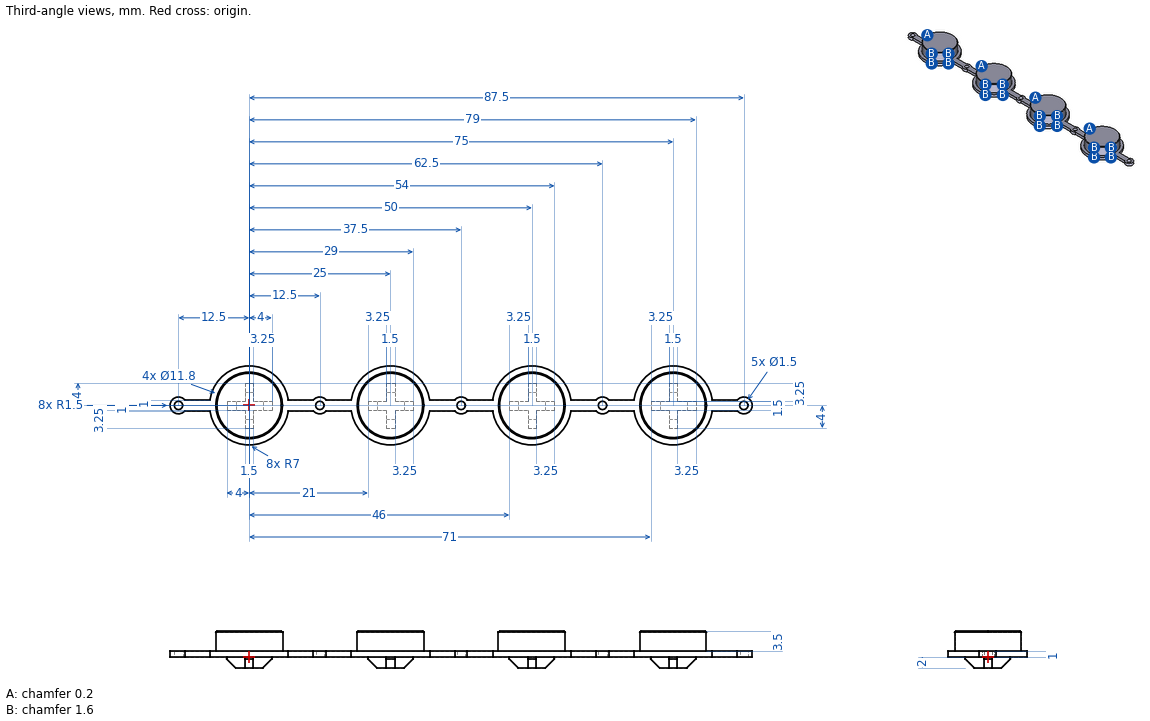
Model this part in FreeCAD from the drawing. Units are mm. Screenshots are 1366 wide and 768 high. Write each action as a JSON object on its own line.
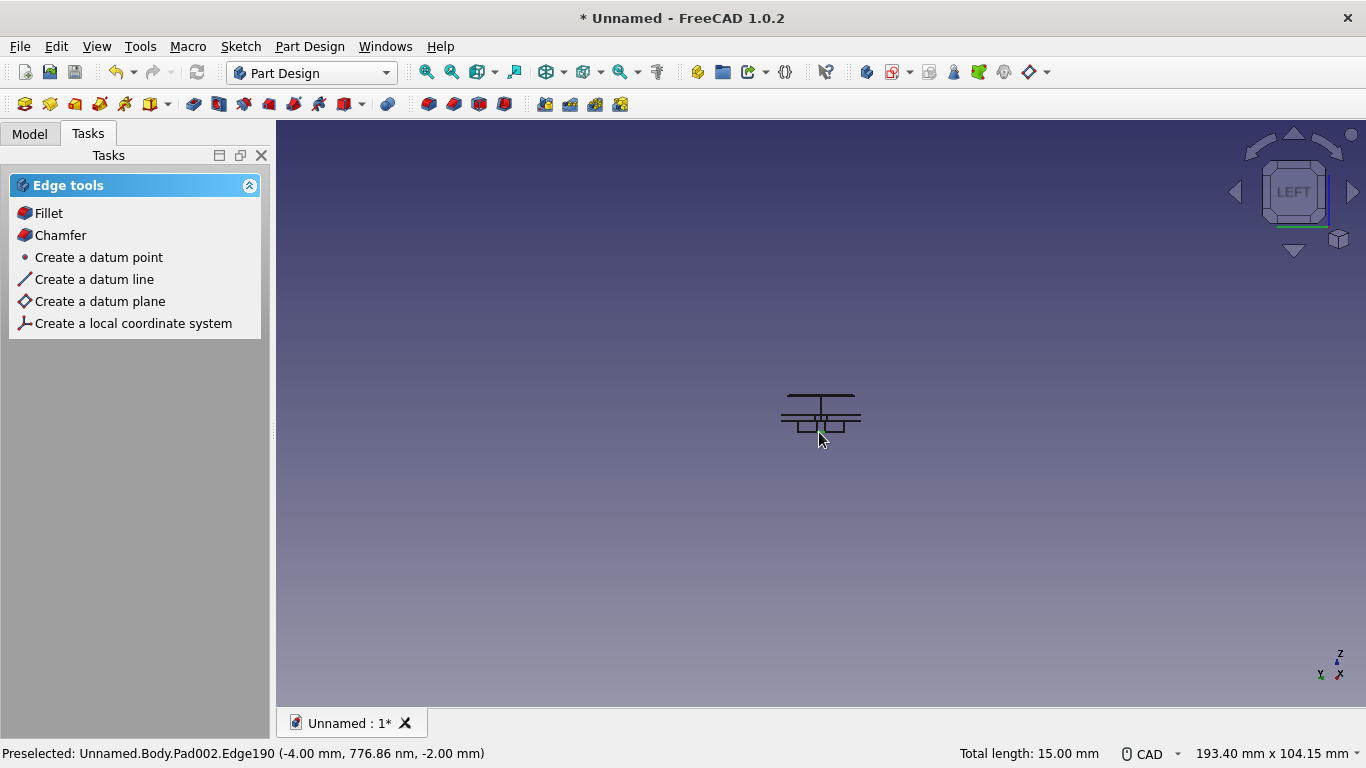
{"action": "key", "text": "0"}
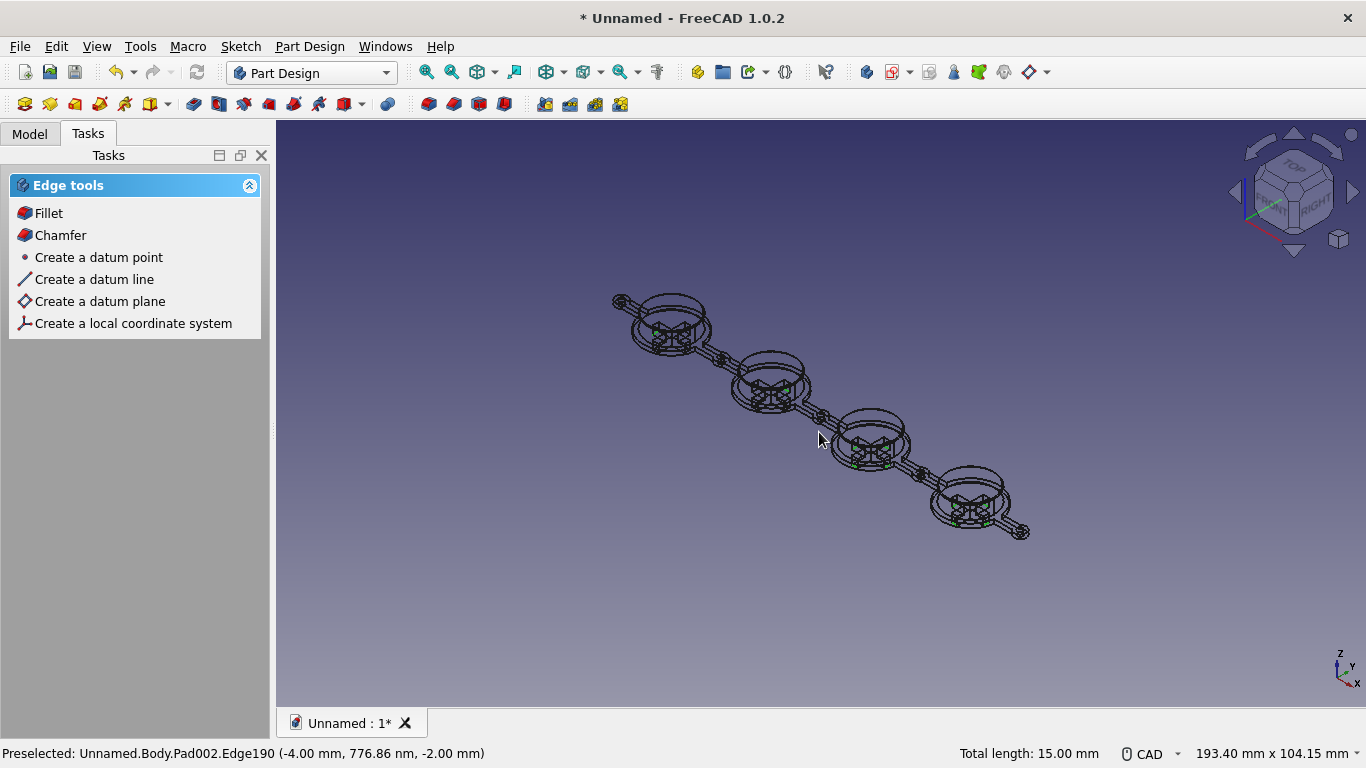
{"action": "scroll", "coordinate": [755, 389], "scroll_direction": "up", "scroll_amount": 8}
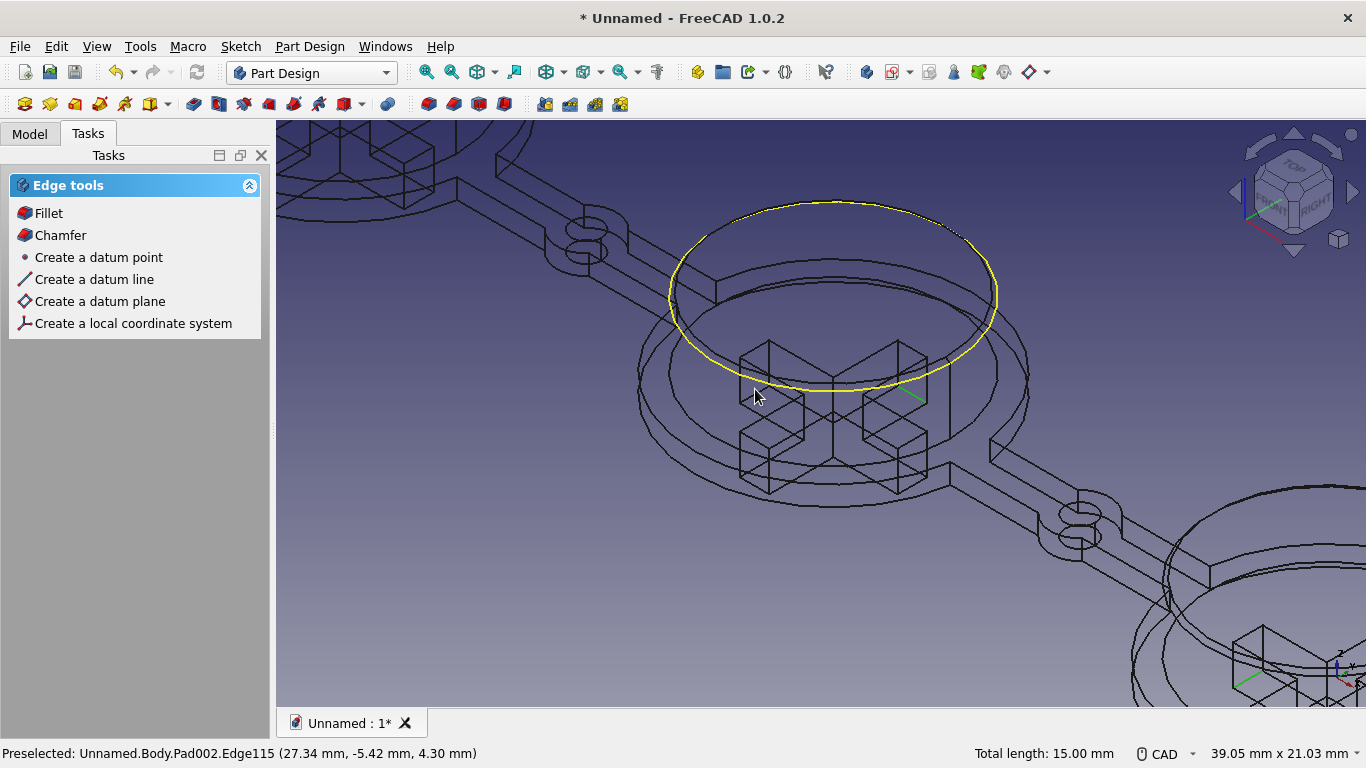
{"action": "left_click", "coordinate": [754, 394], "text": "ctrl"}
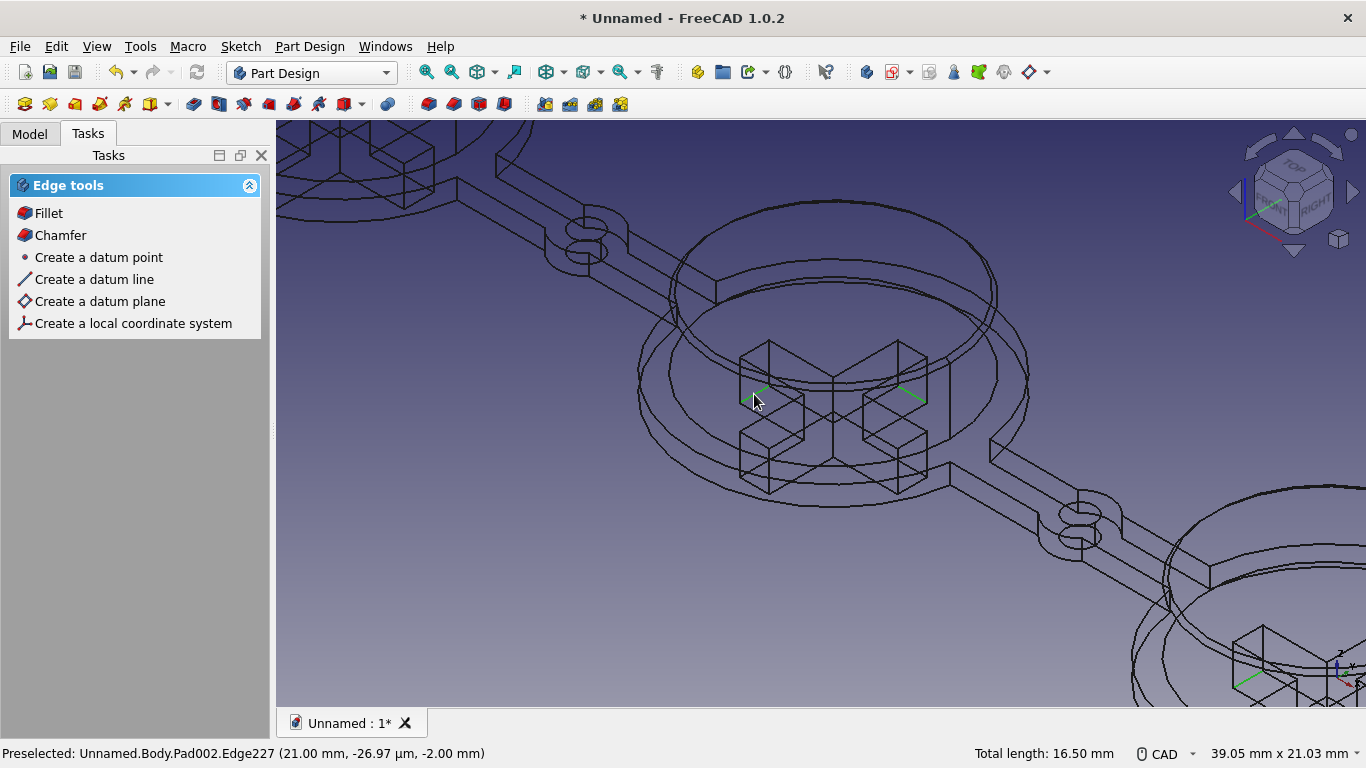
{"action": "left_click", "coordinate": [912, 485], "text": "ctrl"}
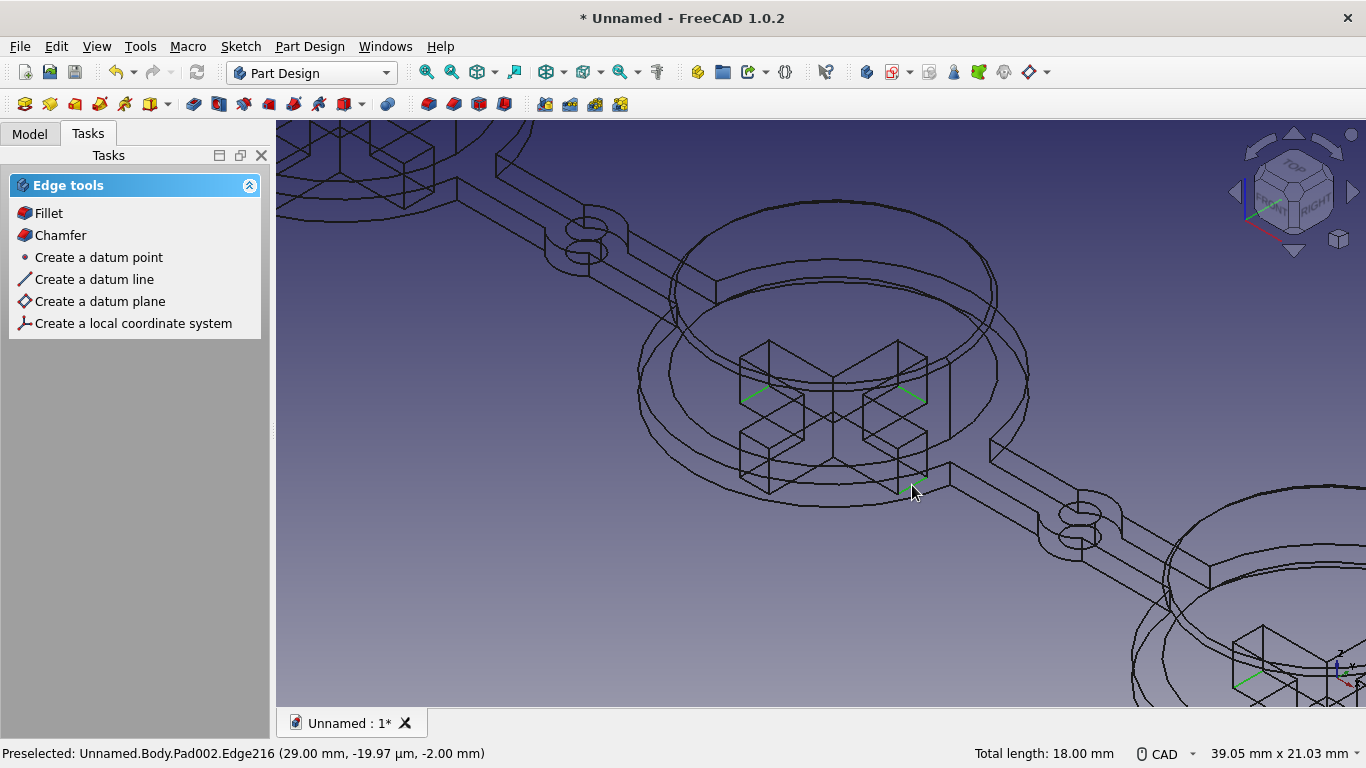
{"action": "left_click", "coordinate": [754, 485], "text": "ctrl"}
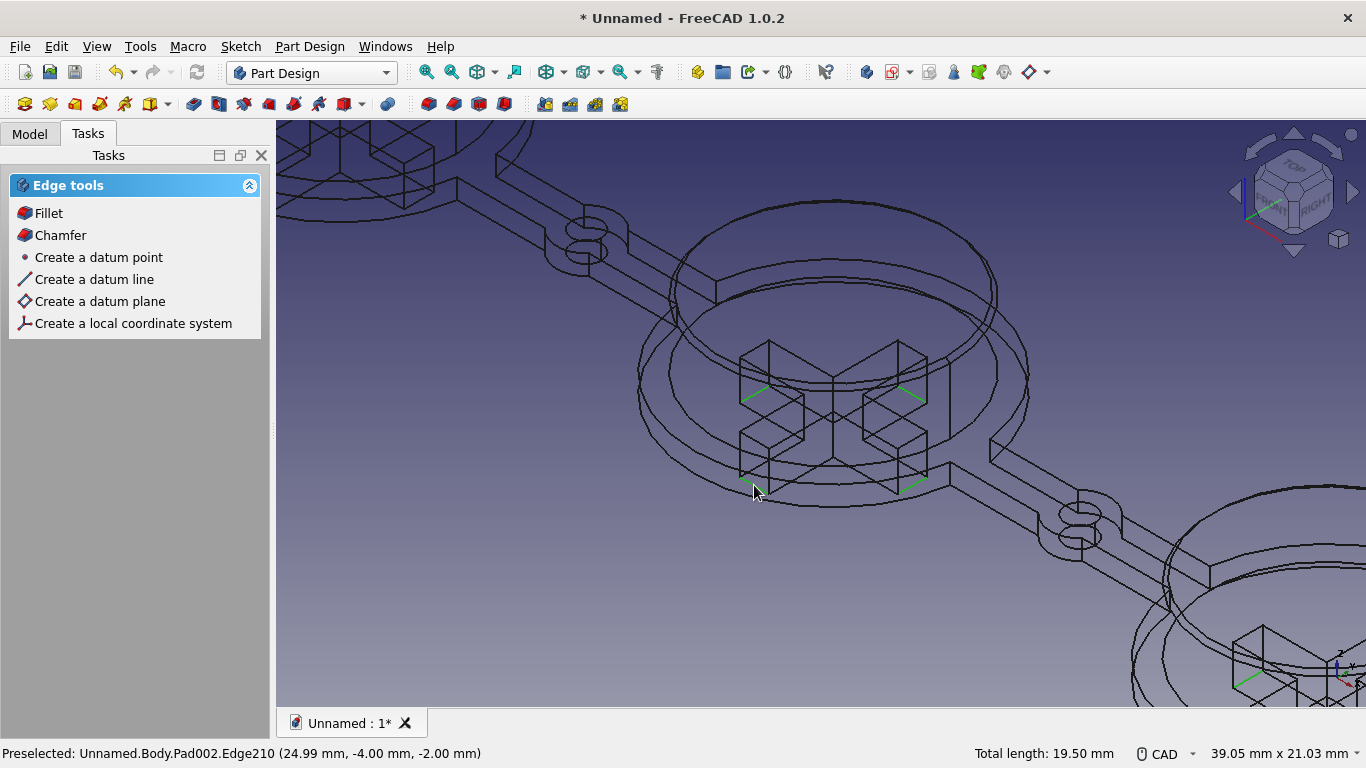
{"action": "left_click", "coordinate": [419, 200], "text": "ctrl"}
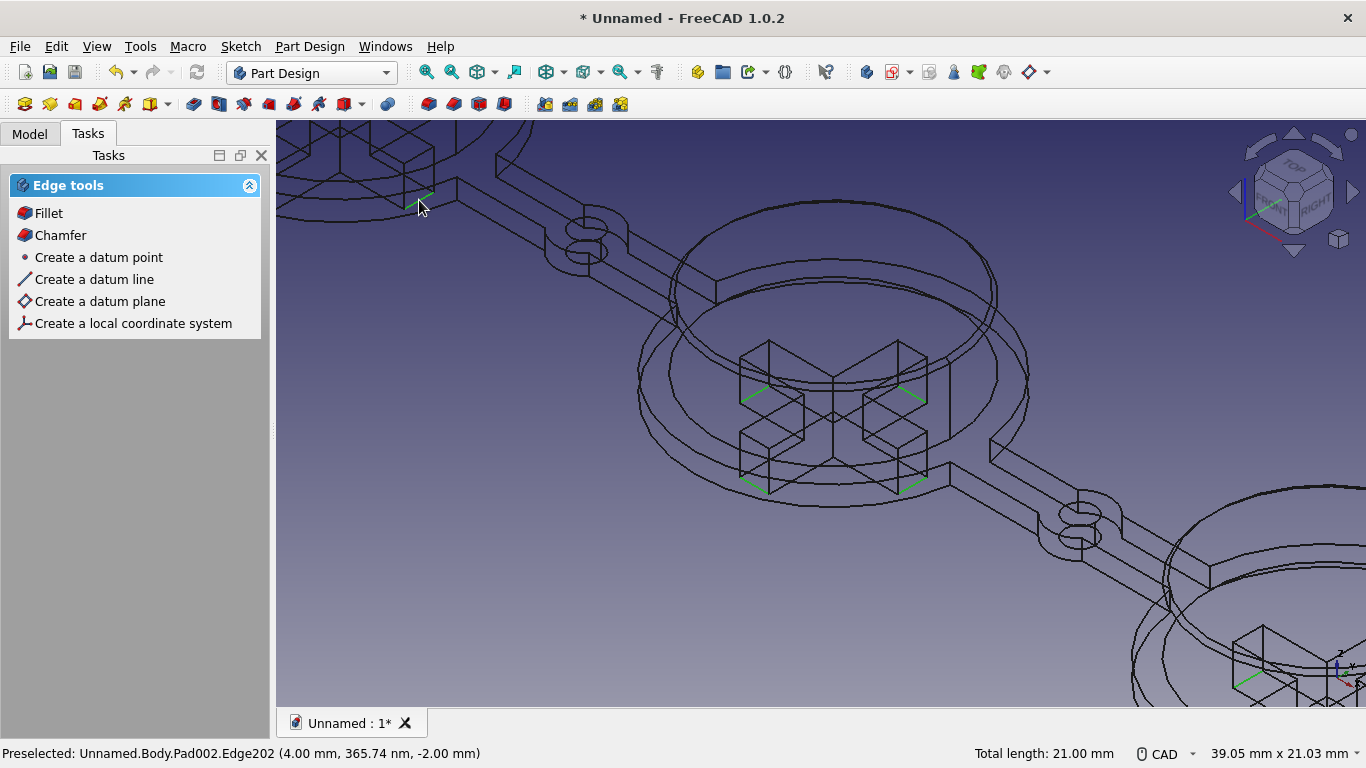
{"action": "key", "text": "v f"}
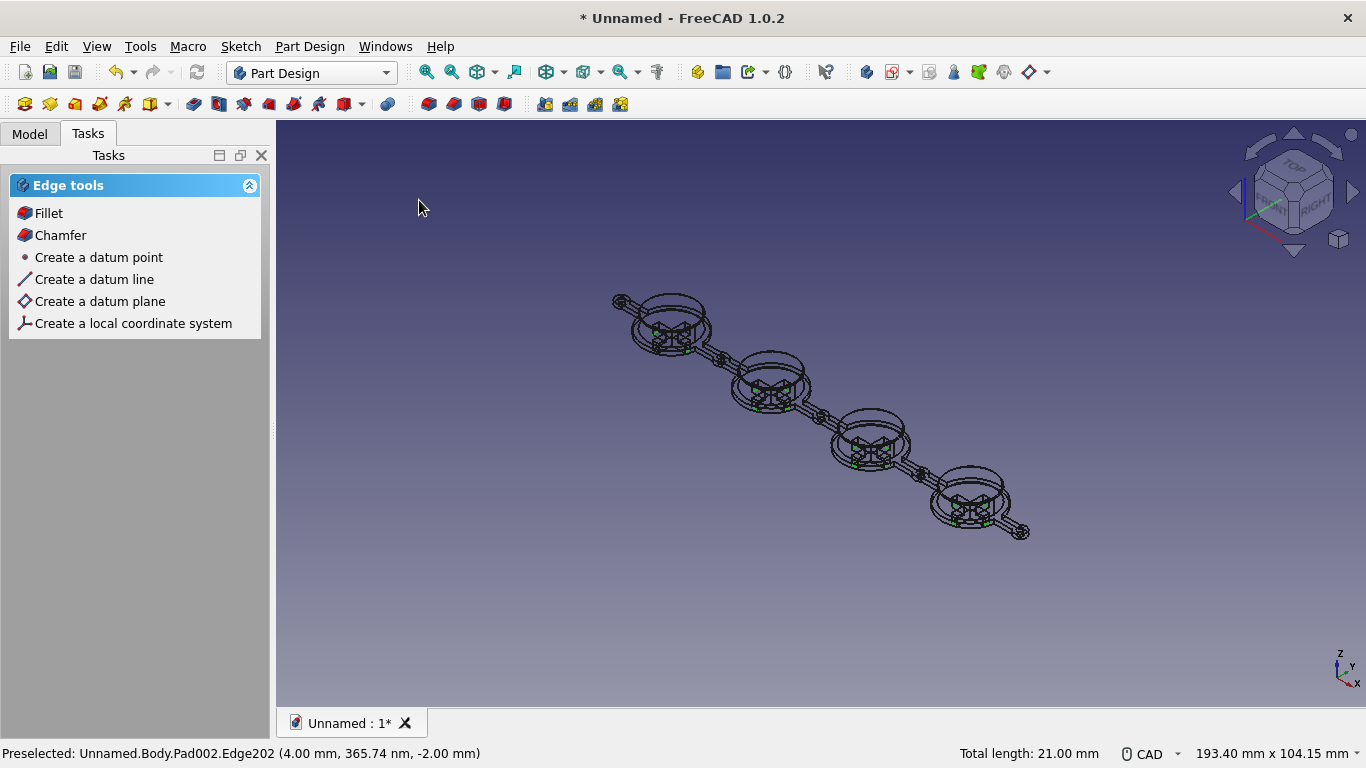
{"action": "key", "text": "2"}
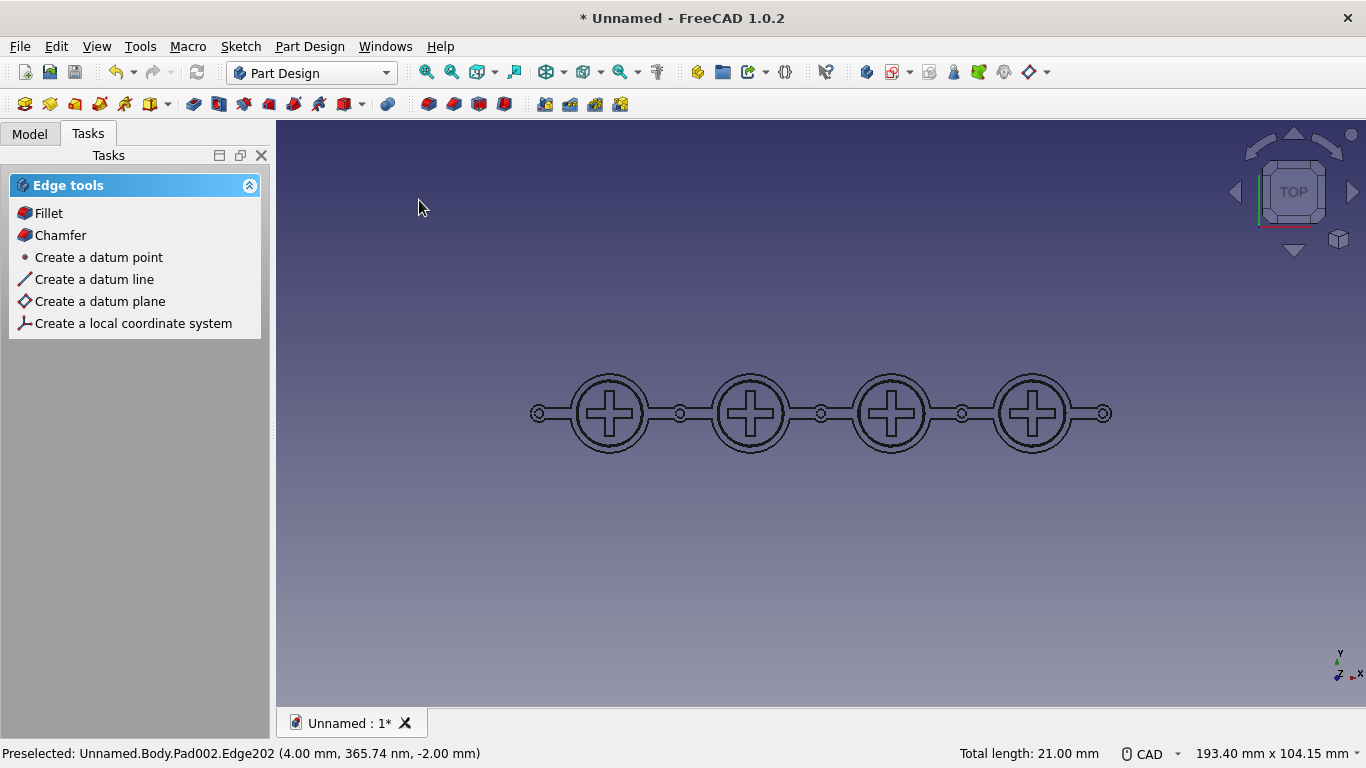
{"action": "scroll", "coordinate": [610, 390], "scroll_direction": "up", "scroll_amount": 8}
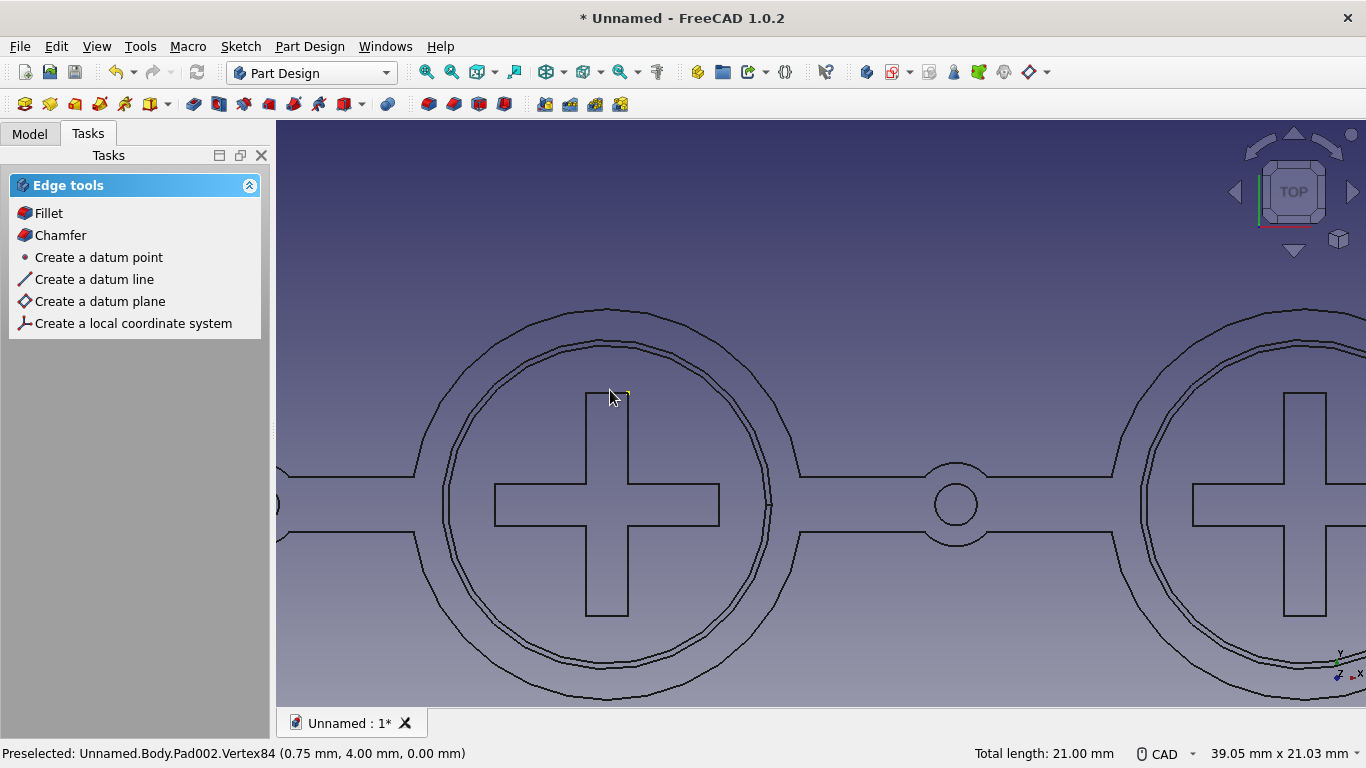
{"action": "left_click", "coordinate": [427, 72]}